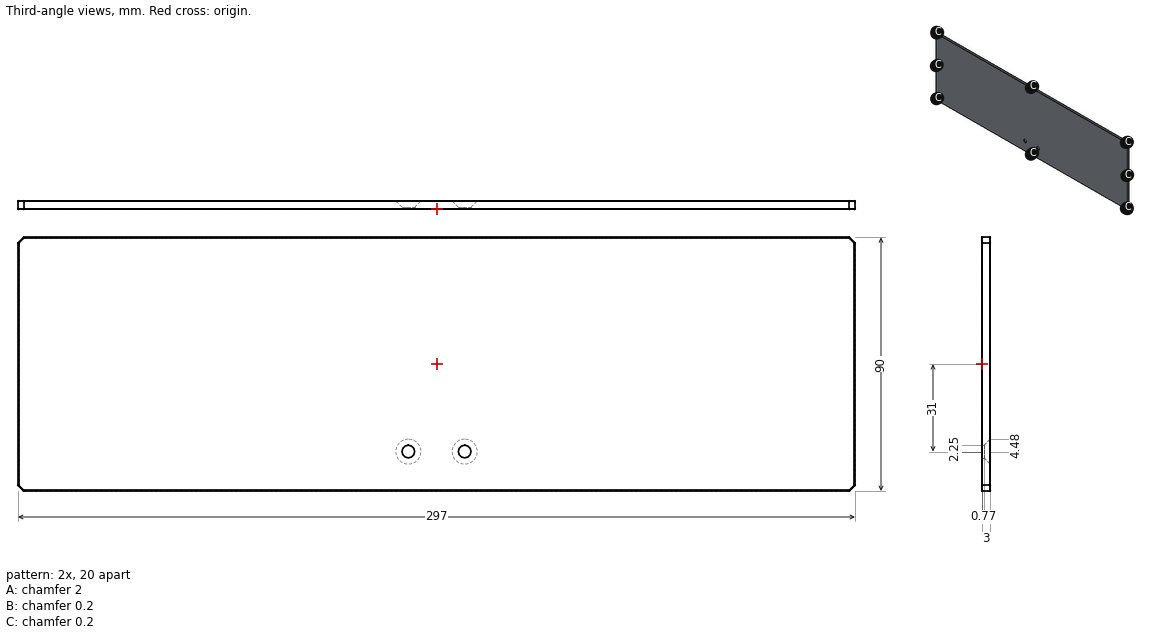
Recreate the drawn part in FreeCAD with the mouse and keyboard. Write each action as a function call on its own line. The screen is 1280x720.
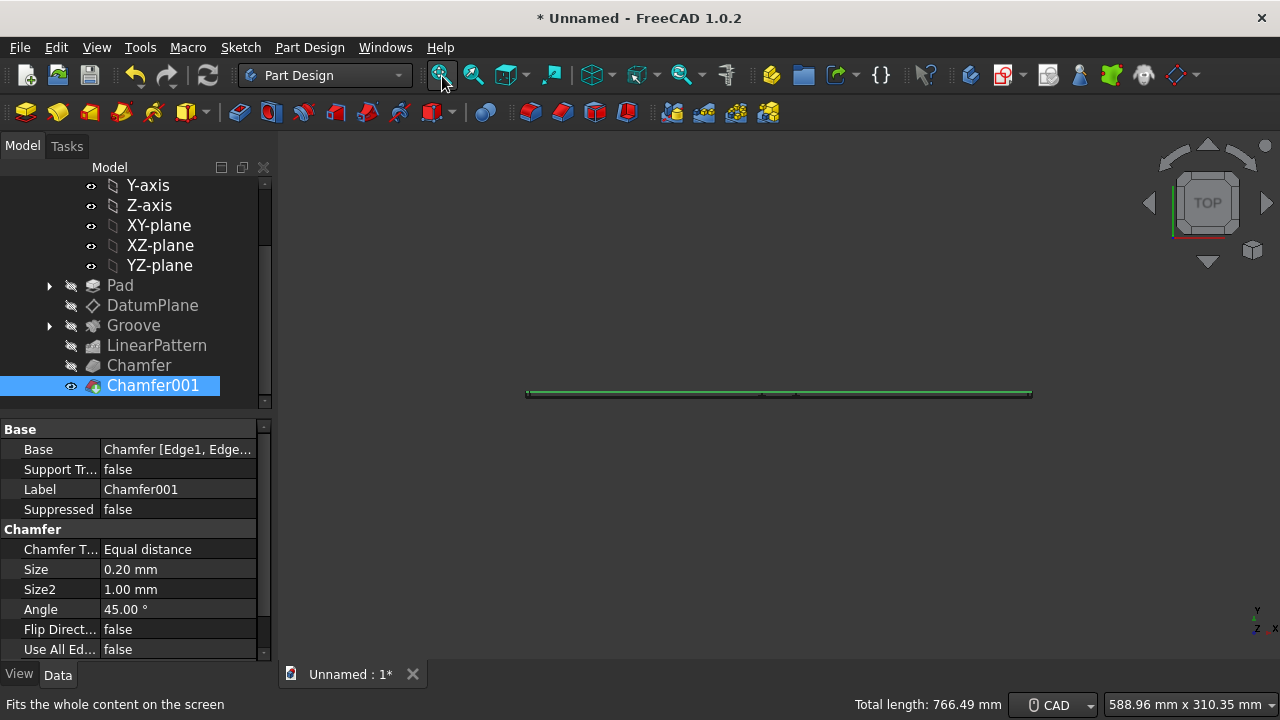
key(1)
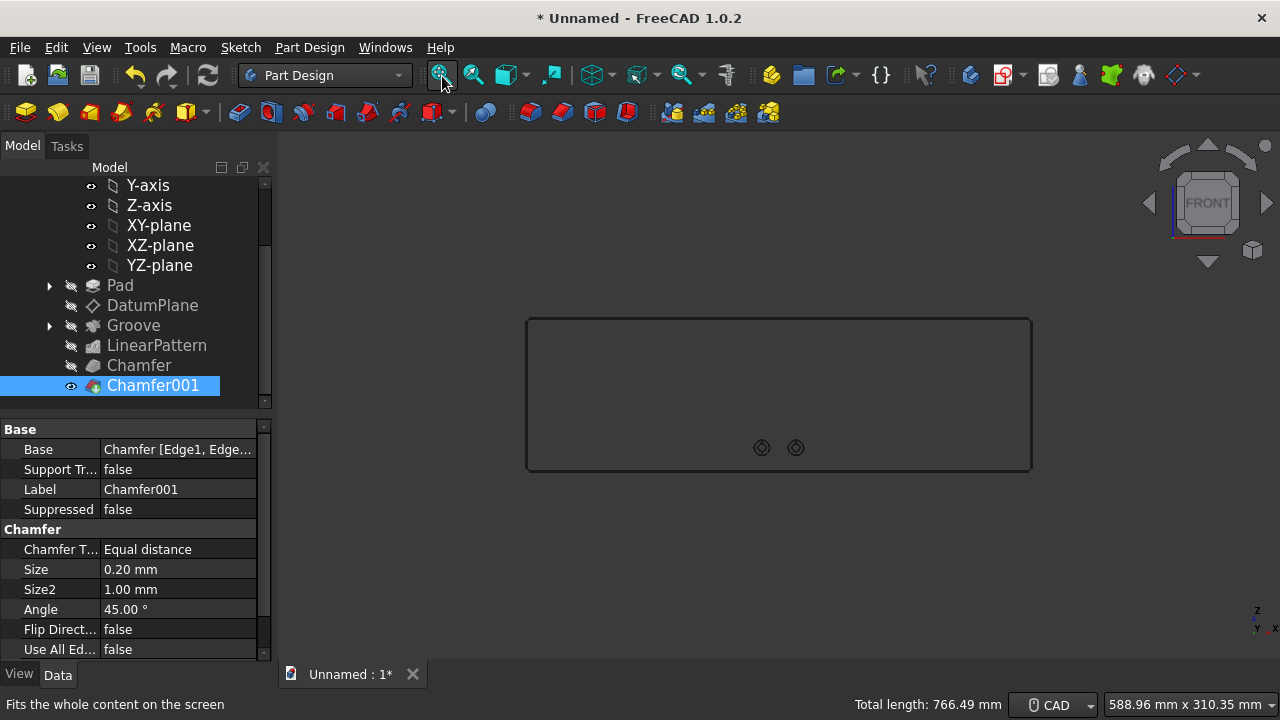
scroll(1030, 469, up, 11)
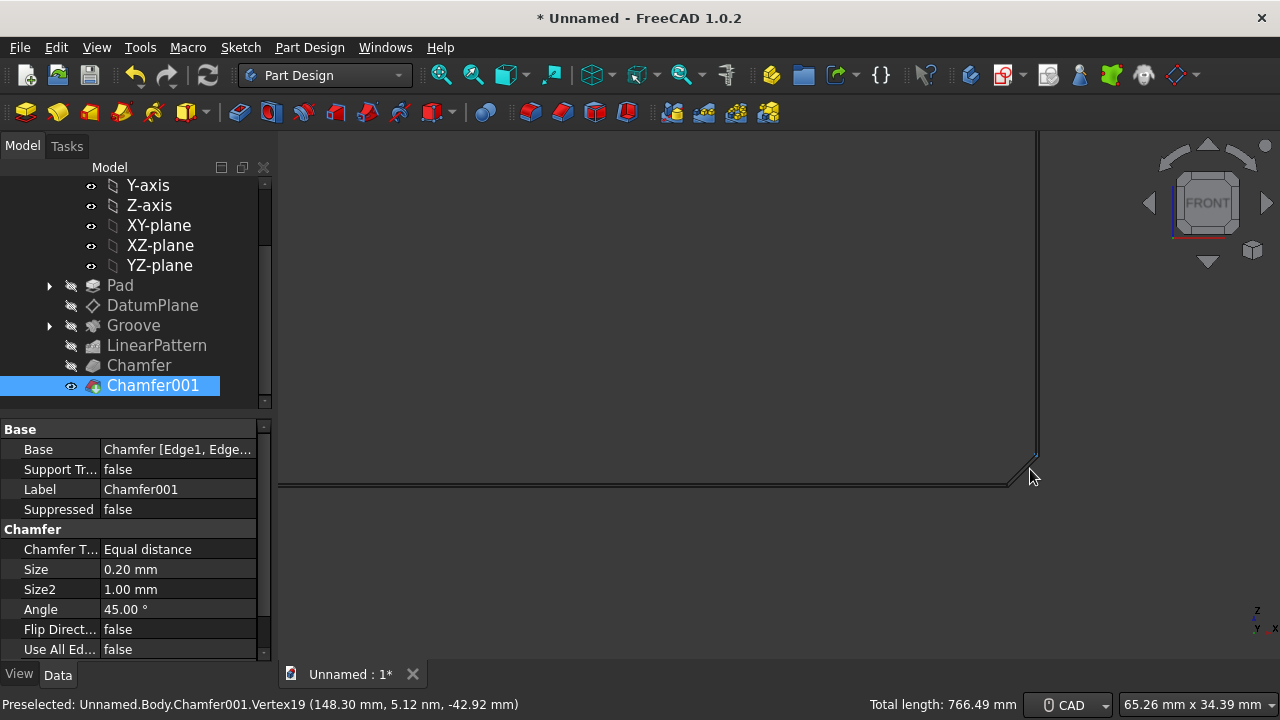
key(v)
key(f)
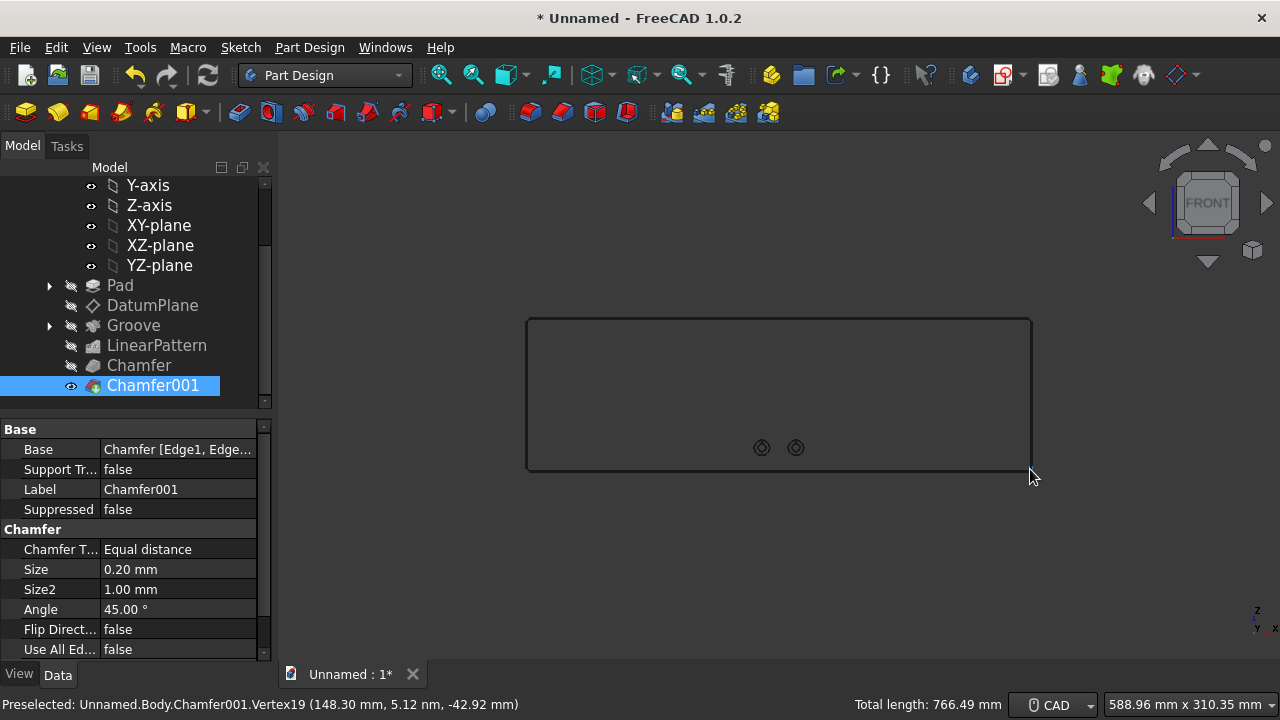
key(3)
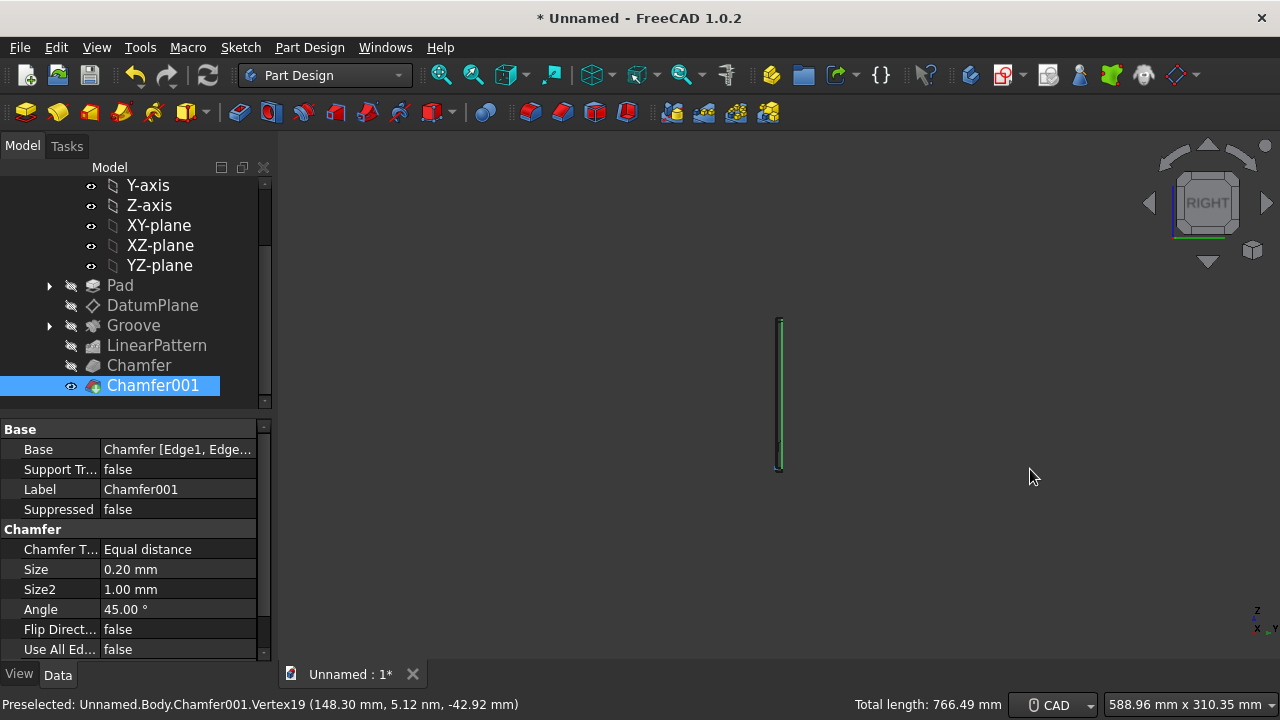
key(v)
key(f)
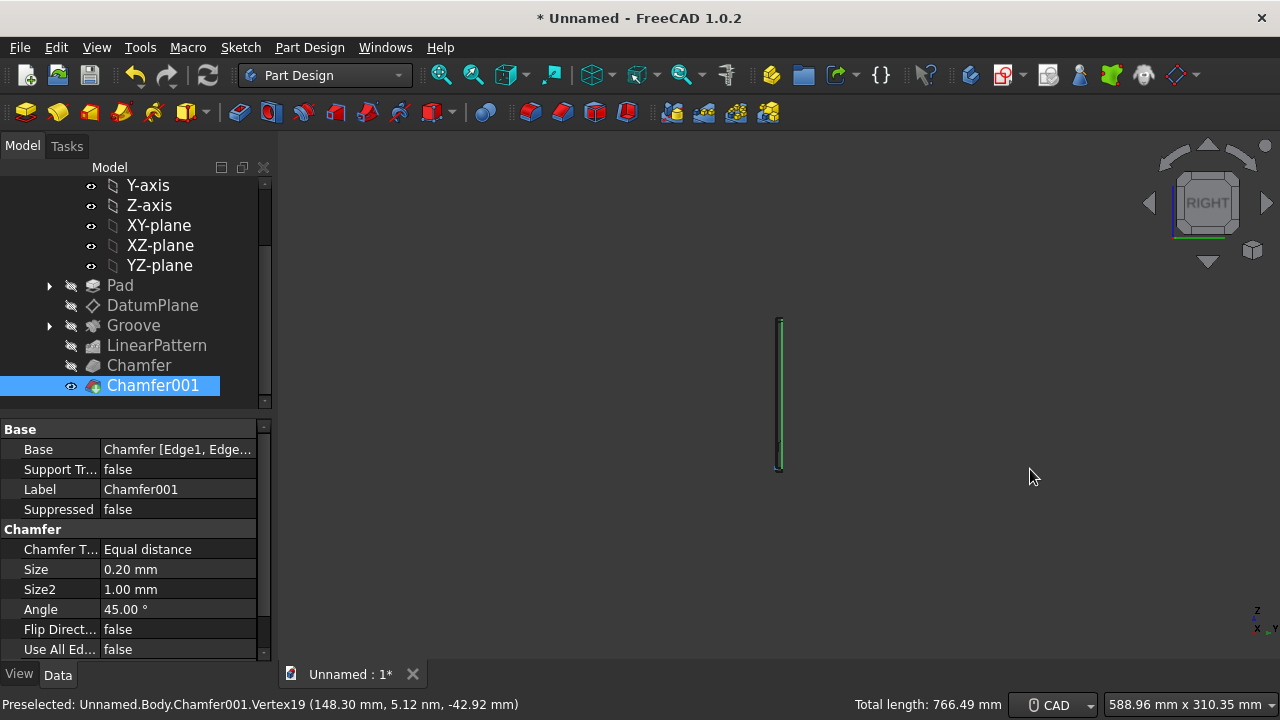
scroll(782, 469, up, 11)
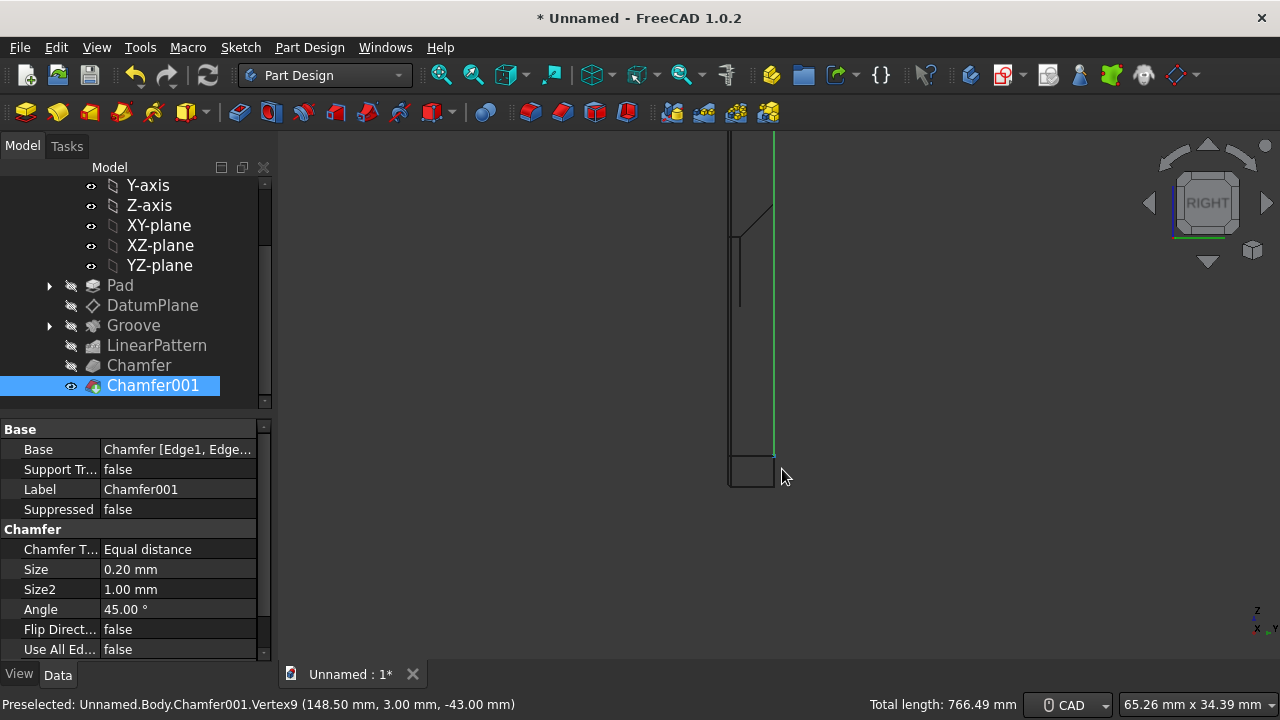
click(774, 471, ctrl)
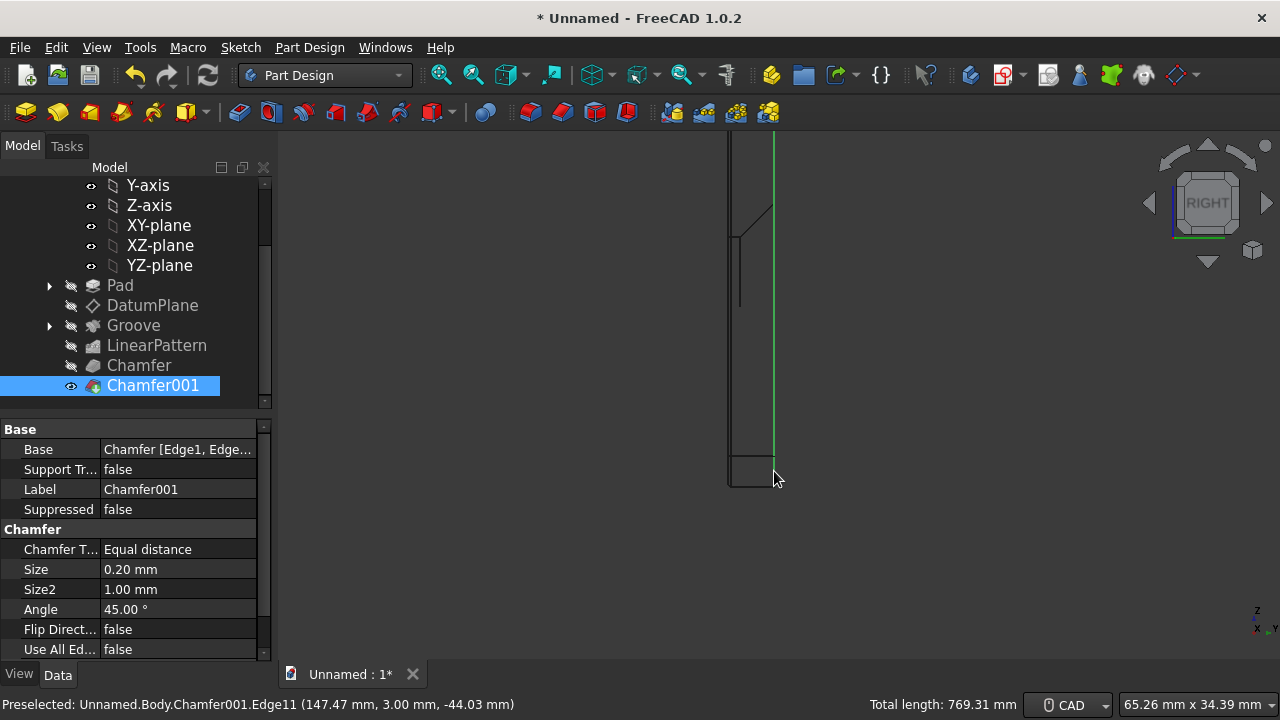
key(v)
key(1)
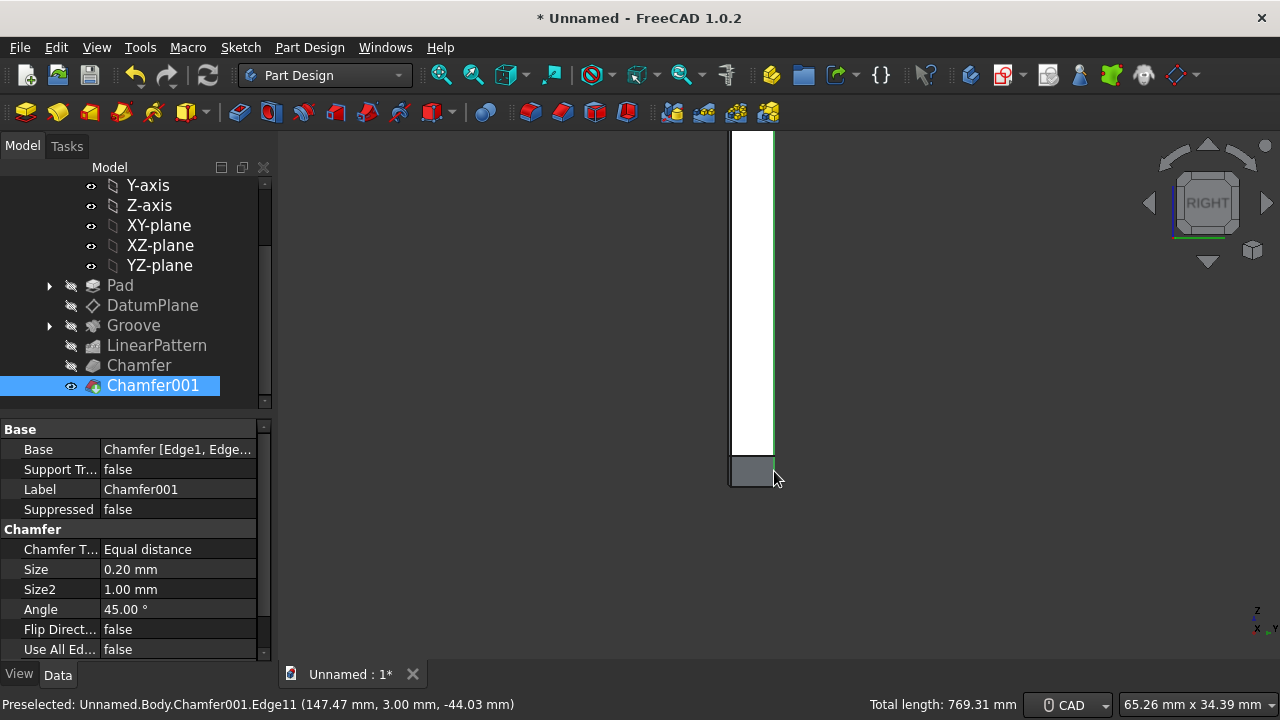
click(564, 112)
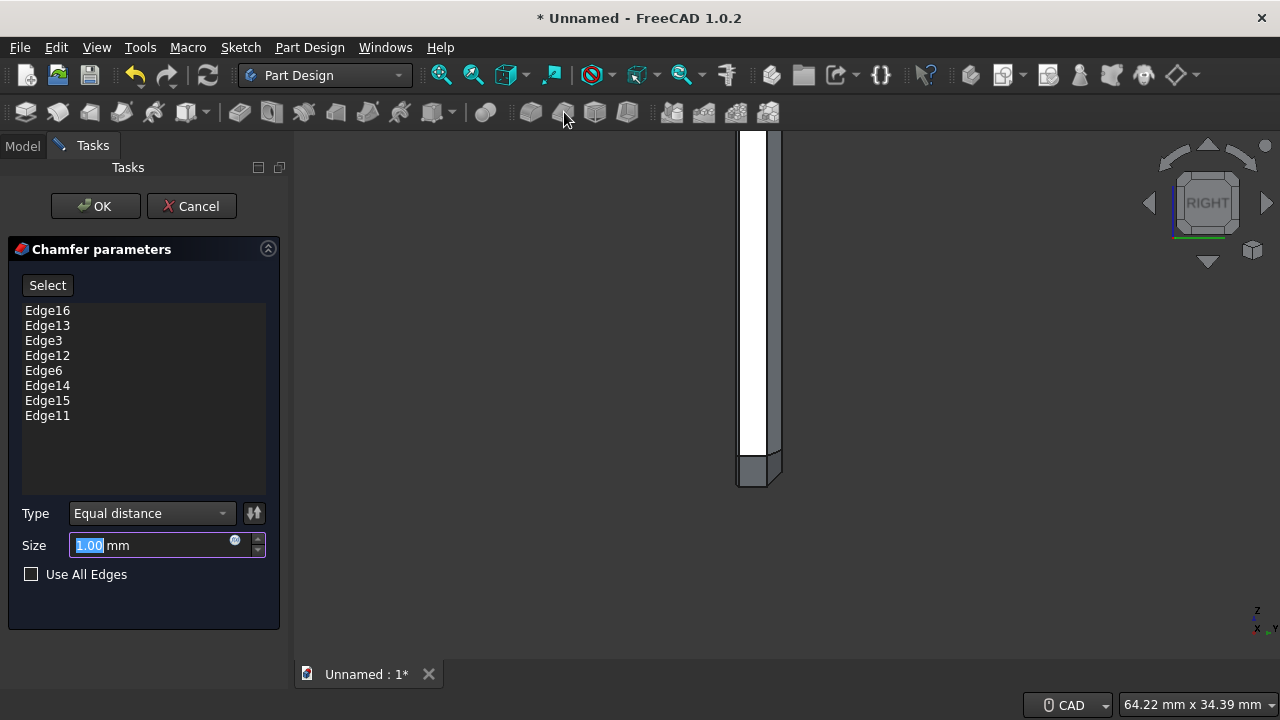
text(0.2)
key(Tab)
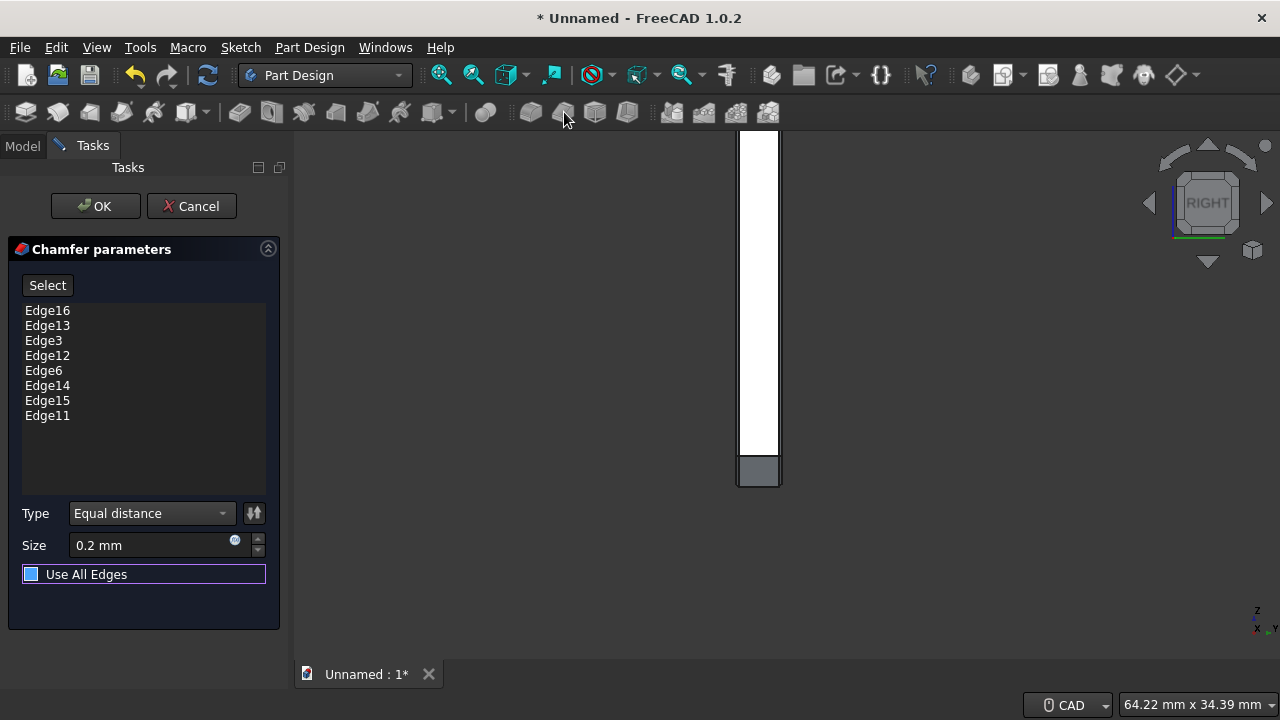
click(96, 206)